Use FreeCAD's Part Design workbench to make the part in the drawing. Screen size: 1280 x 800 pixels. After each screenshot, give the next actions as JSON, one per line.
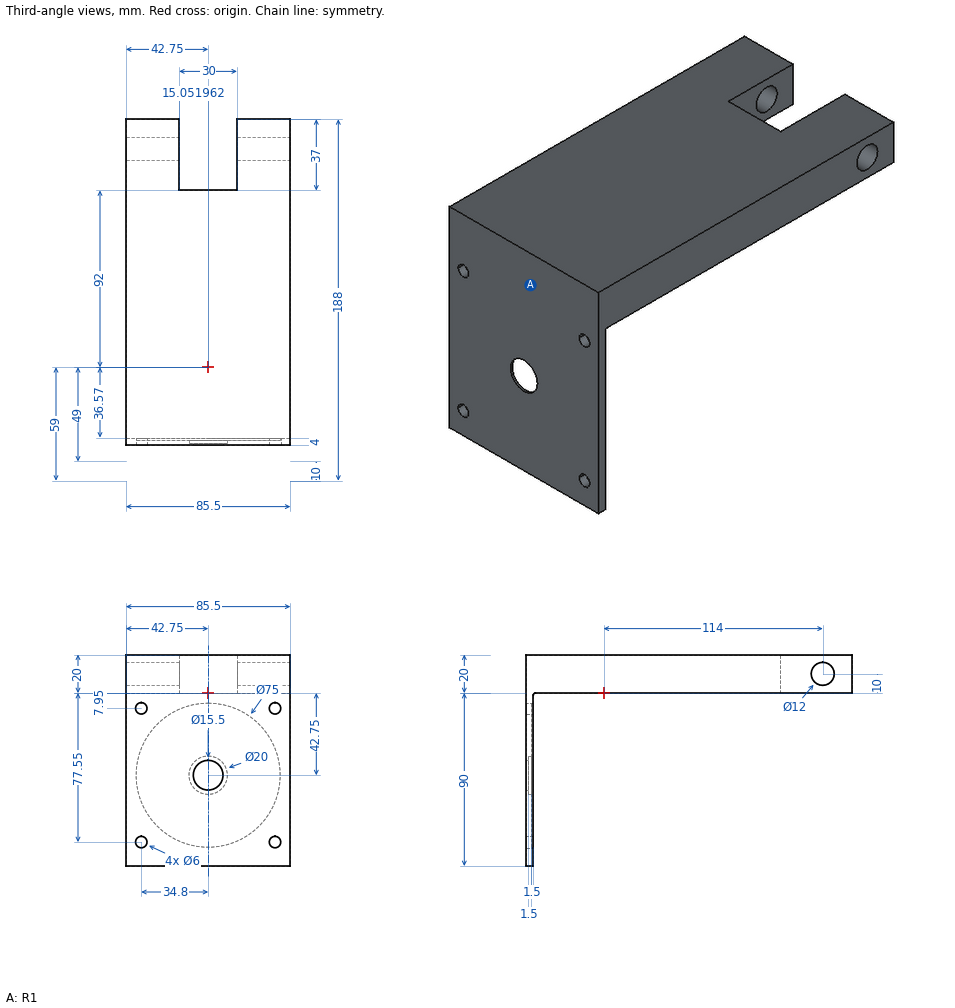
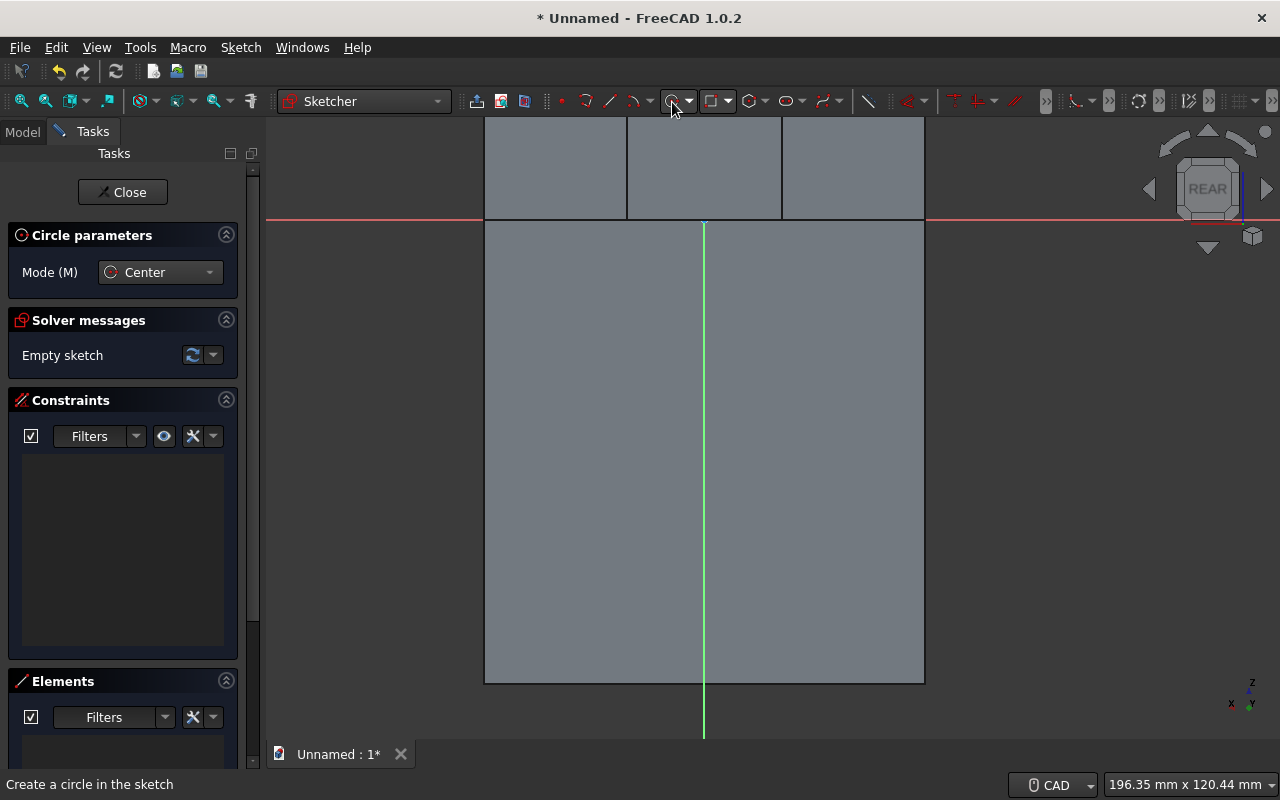
{"action": "scroll", "coordinate": [884, 620], "scroll_direction": "up", "scroll_amount": 2}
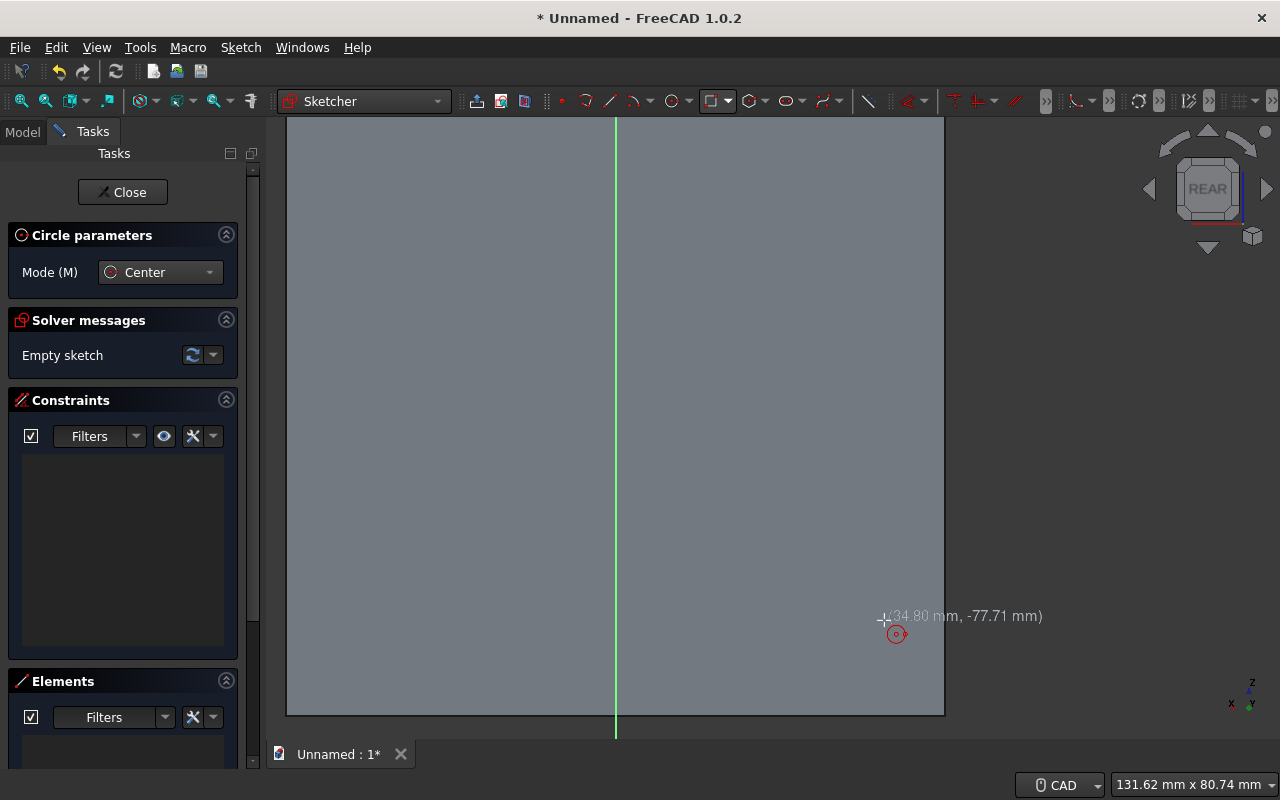
{"action": "left_click", "coordinate": [884, 620]}
{"action": "mouse_move", "coordinate": [900, 603]}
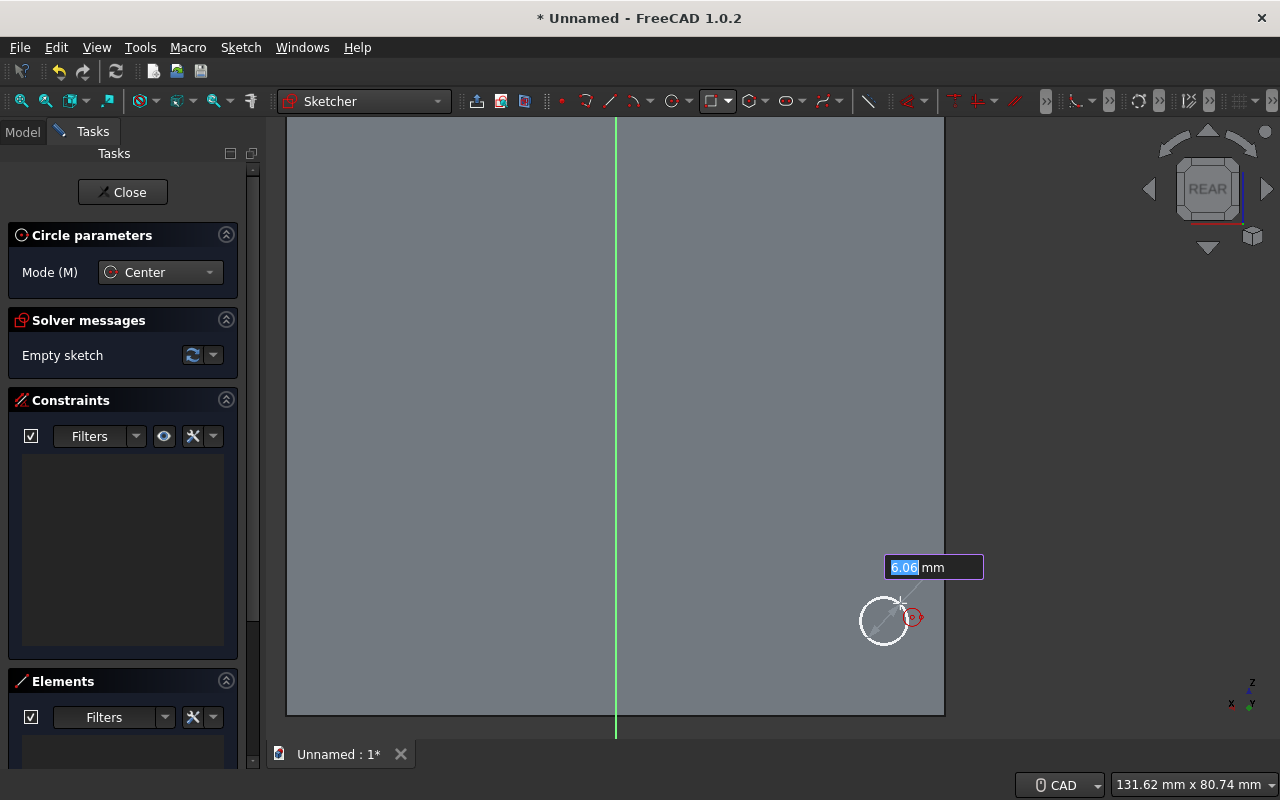
{"action": "type", "text": "6"}
{"action": "key", "text": "Return"}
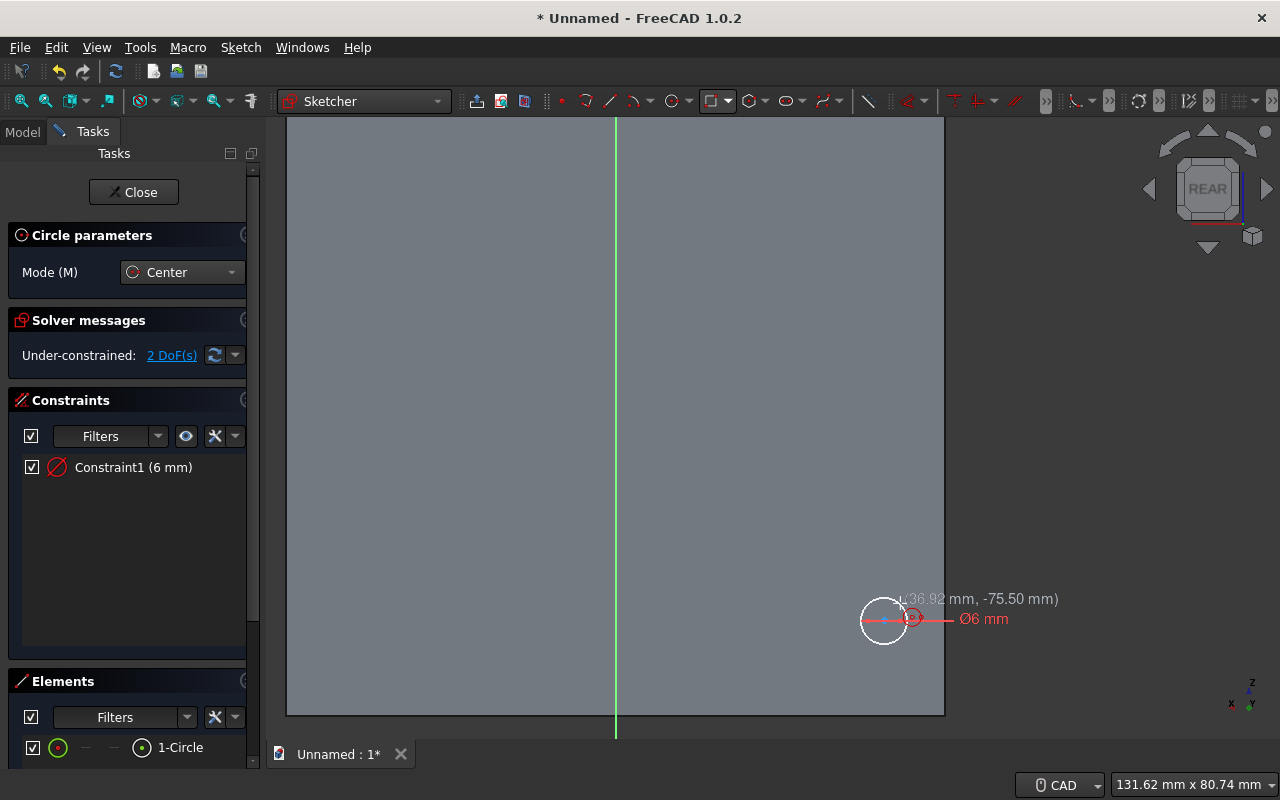
{"action": "left_click", "coordinate": [347, 620]}
{"action": "mouse_move", "coordinate": [364, 603]}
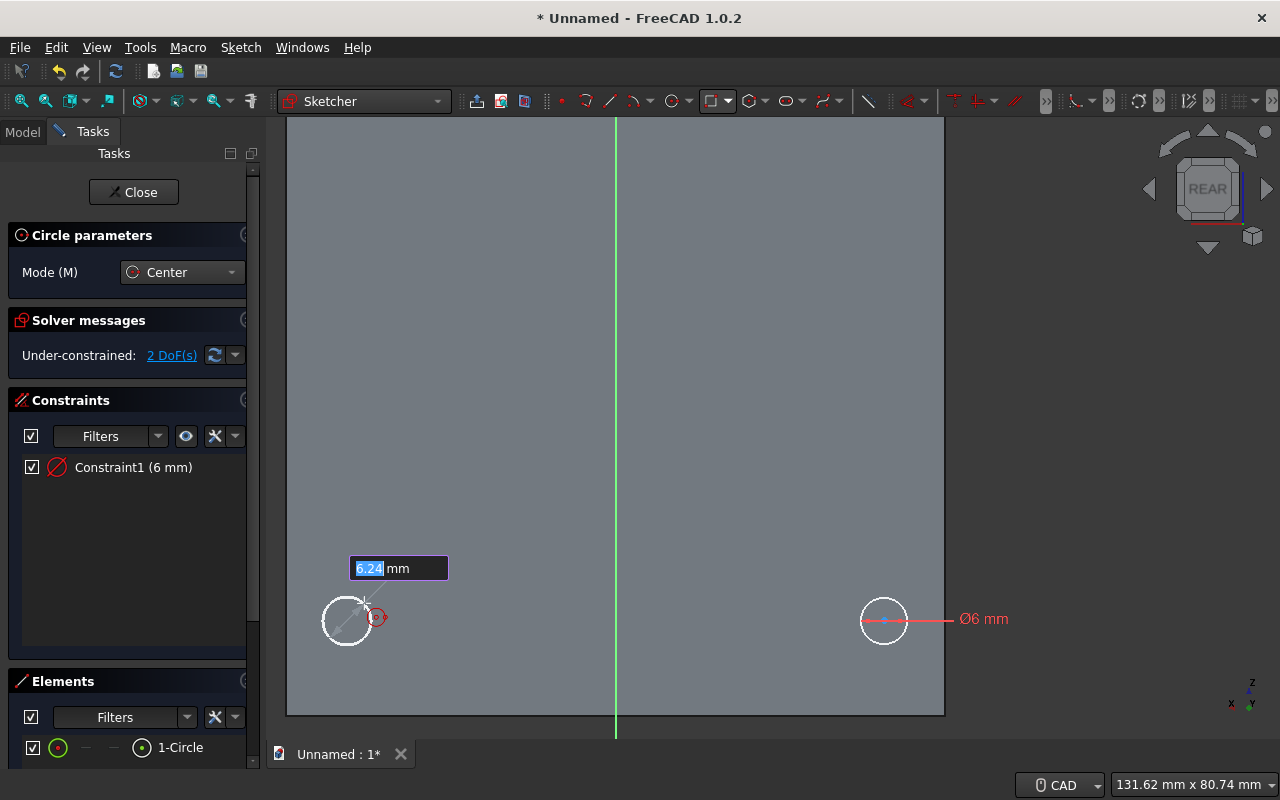
{"action": "type", "text": "6"}
{"action": "key", "text": "Return"}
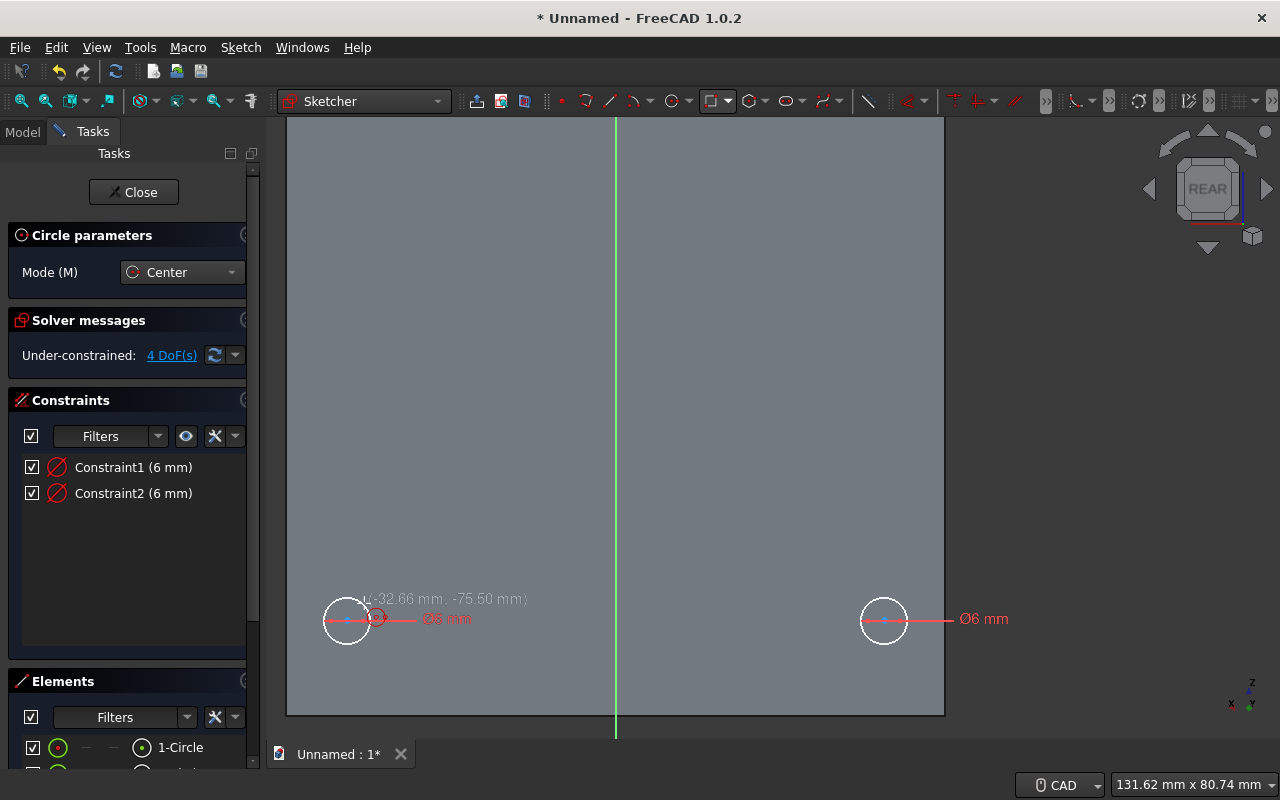
{"action": "scroll", "coordinate": [885, 622], "scroll_direction": "down", "scroll_amount": 2}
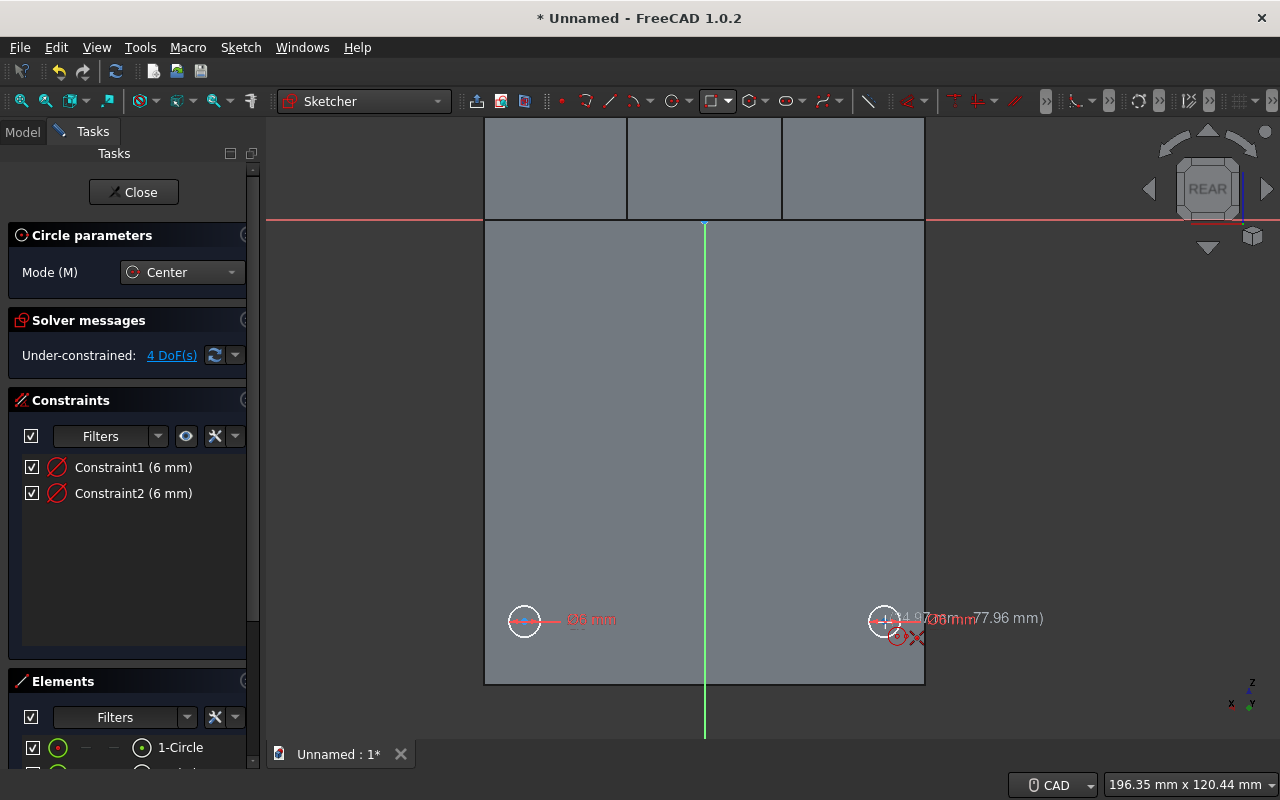
{"action": "scroll", "coordinate": [884, 261], "scroll_direction": "up", "scroll_amount": 2}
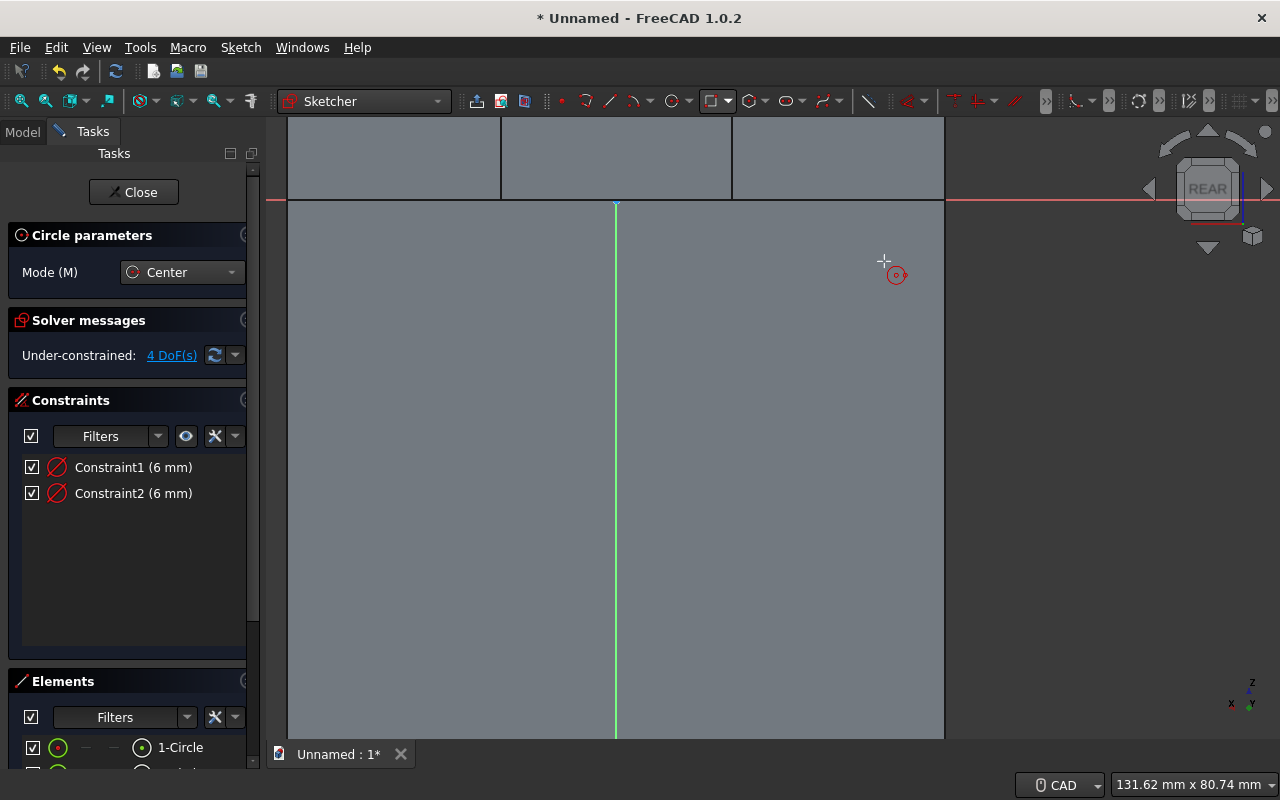
{"action": "left_click", "coordinate": [884, 261]}
{"action": "mouse_move", "coordinate": [901, 245]}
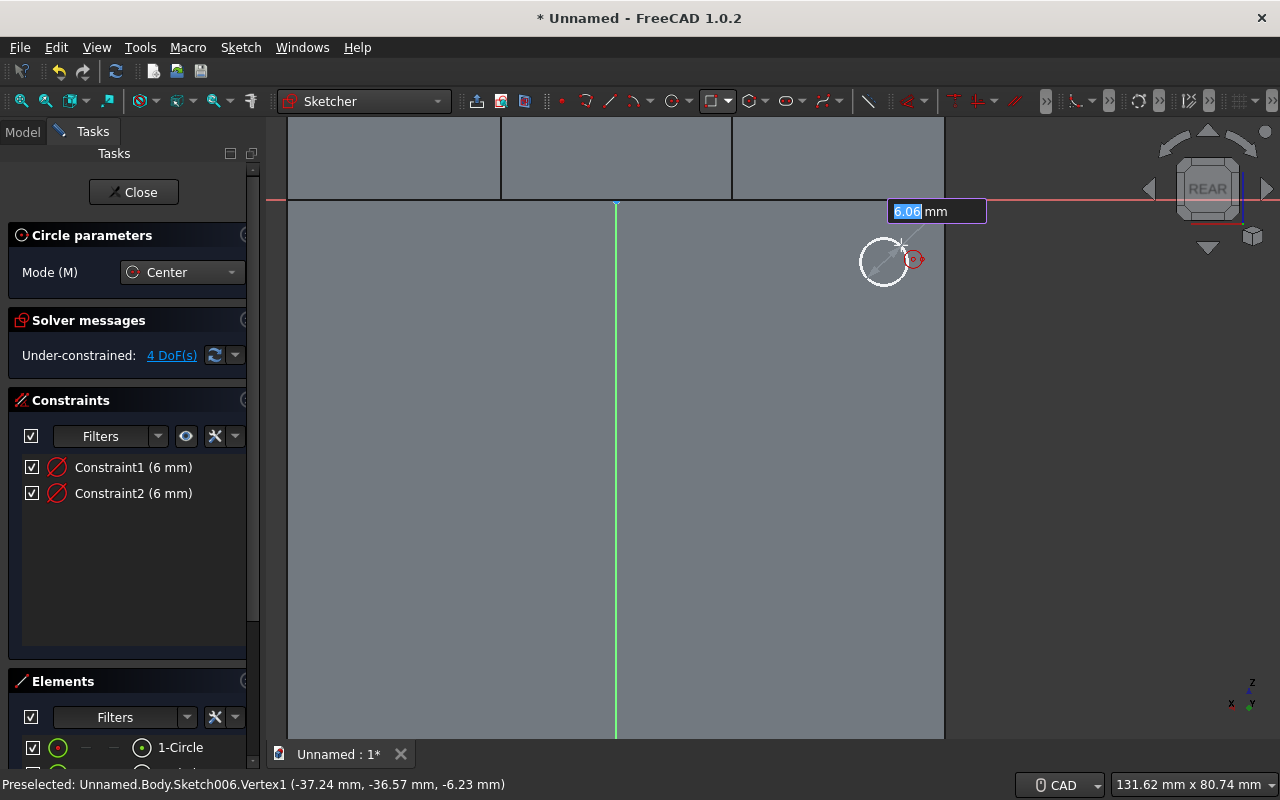
{"action": "type", "text": "6"}
{"action": "key", "text": "Return"}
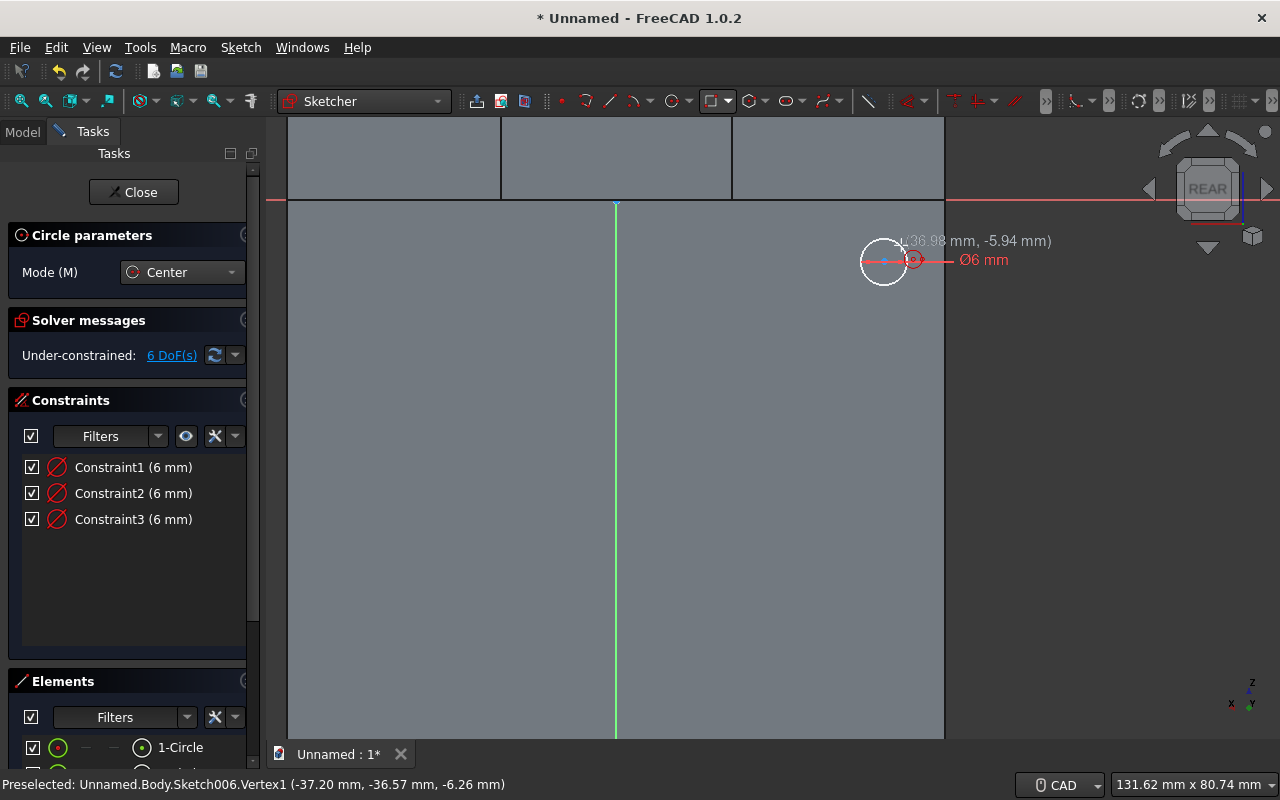
{"action": "left_click", "coordinate": [348, 261]}
{"action": "mouse_move", "coordinate": [364, 245]}